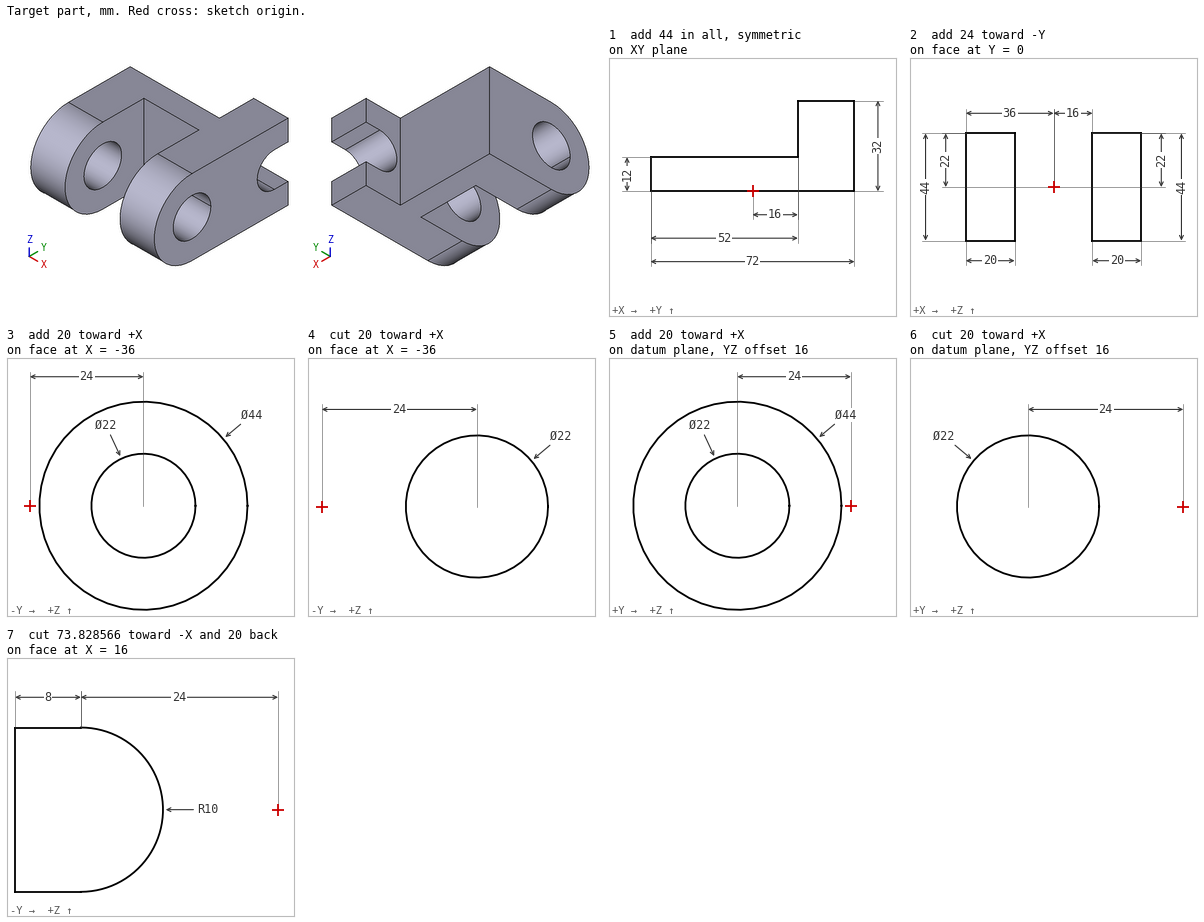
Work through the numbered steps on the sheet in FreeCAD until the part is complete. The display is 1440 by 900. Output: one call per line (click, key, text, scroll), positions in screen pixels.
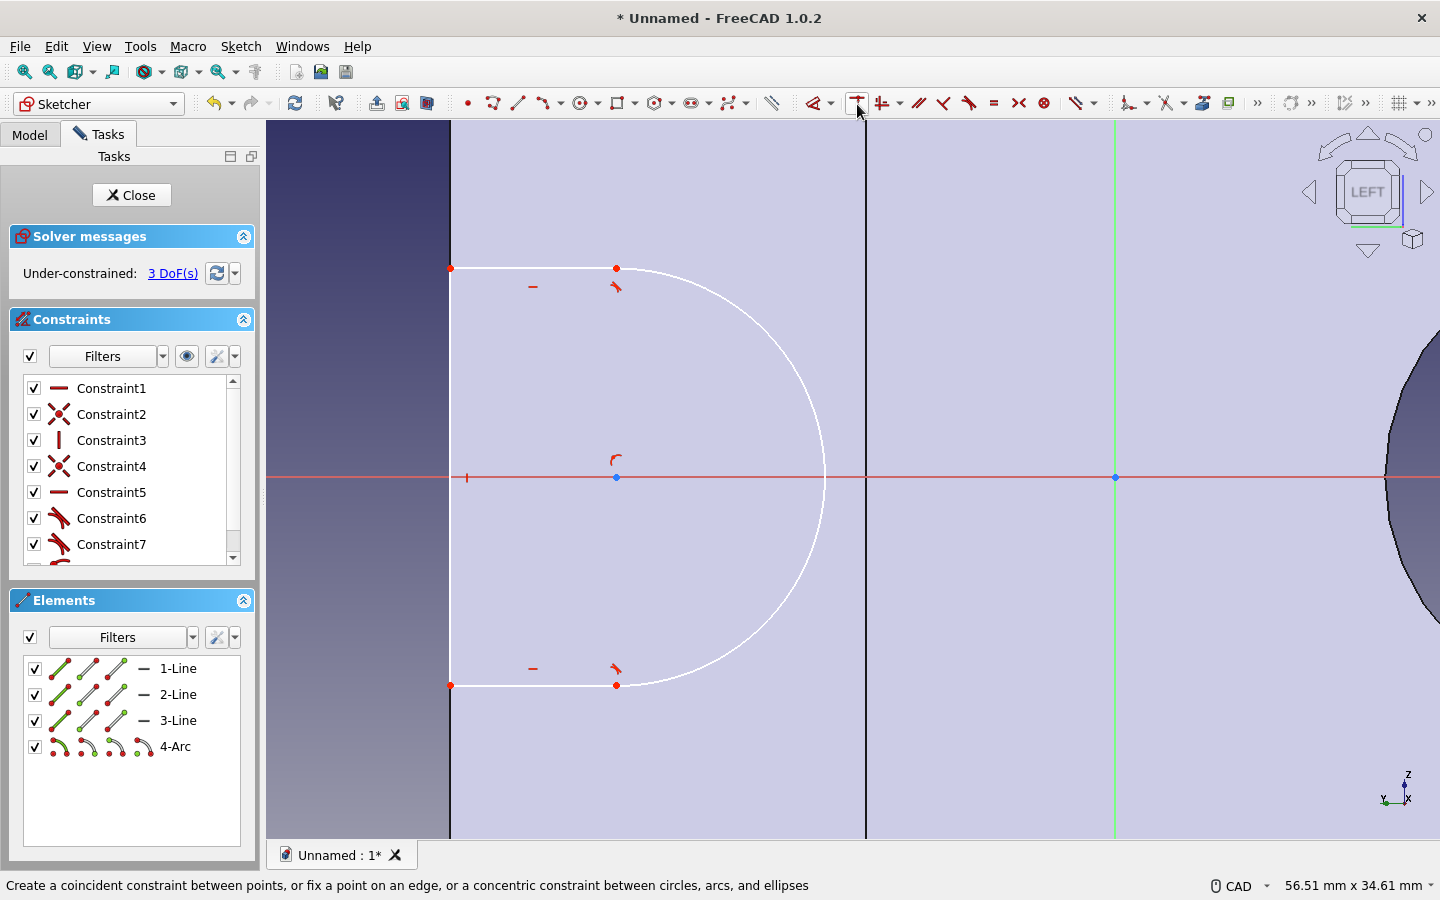
click(812, 104)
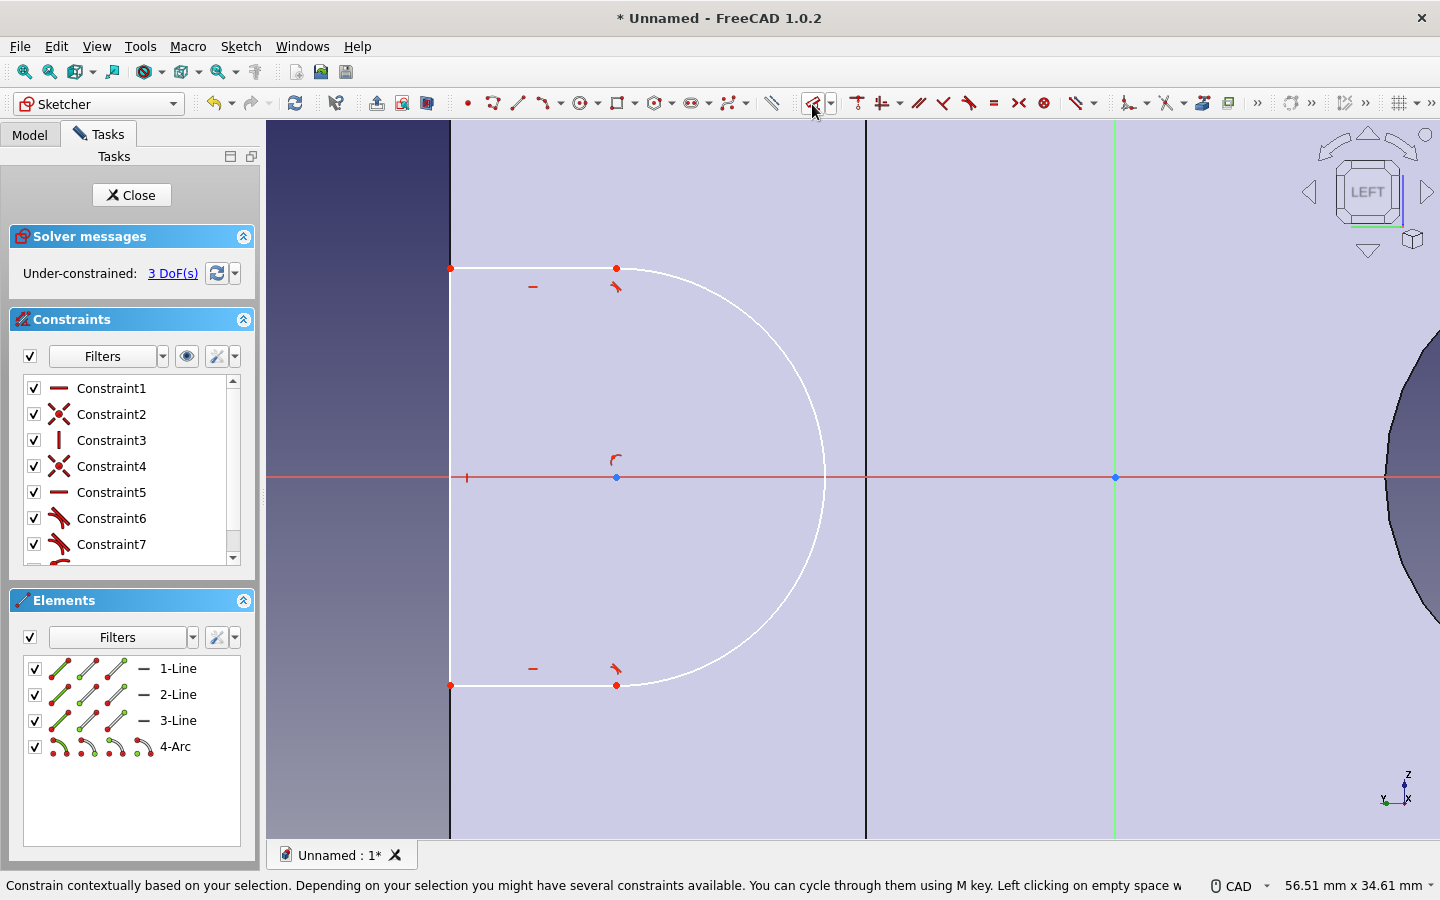
click(785, 600)
click(811, 619)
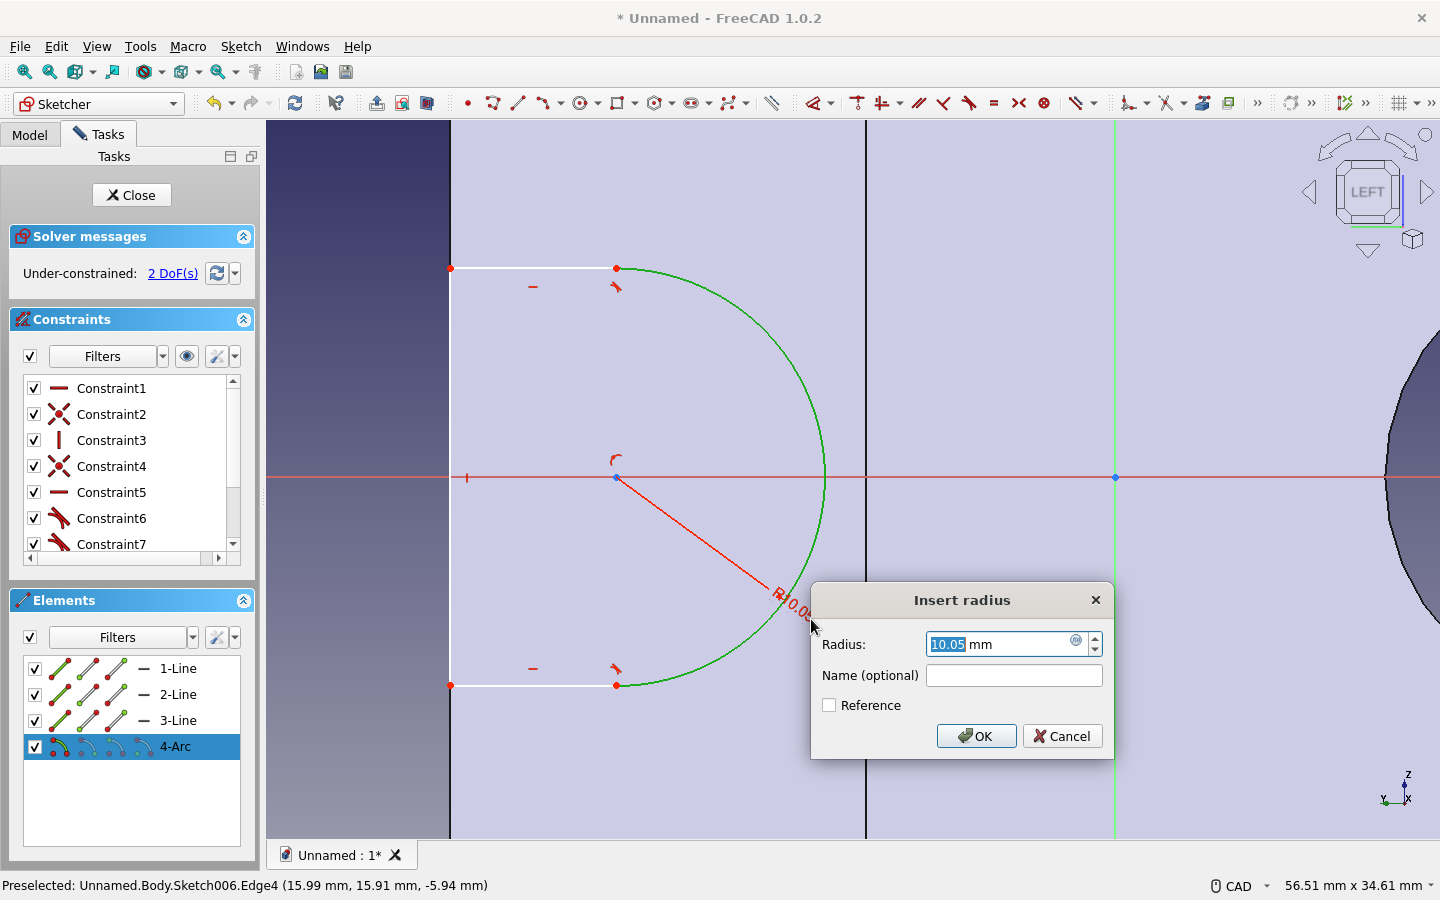
text(10)
key(Return)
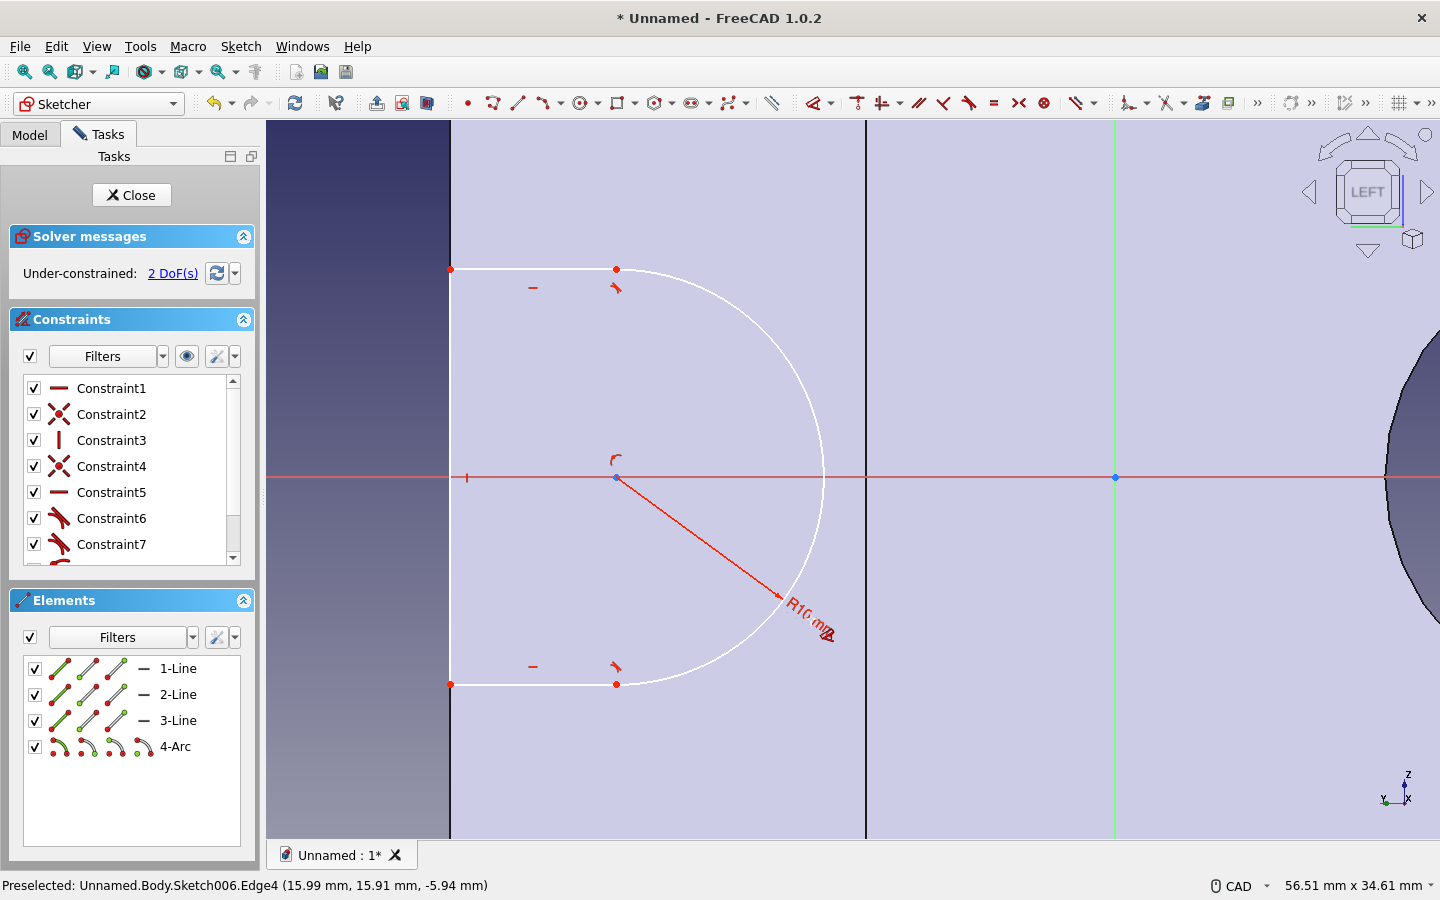
click(566, 269)
click(533, 235)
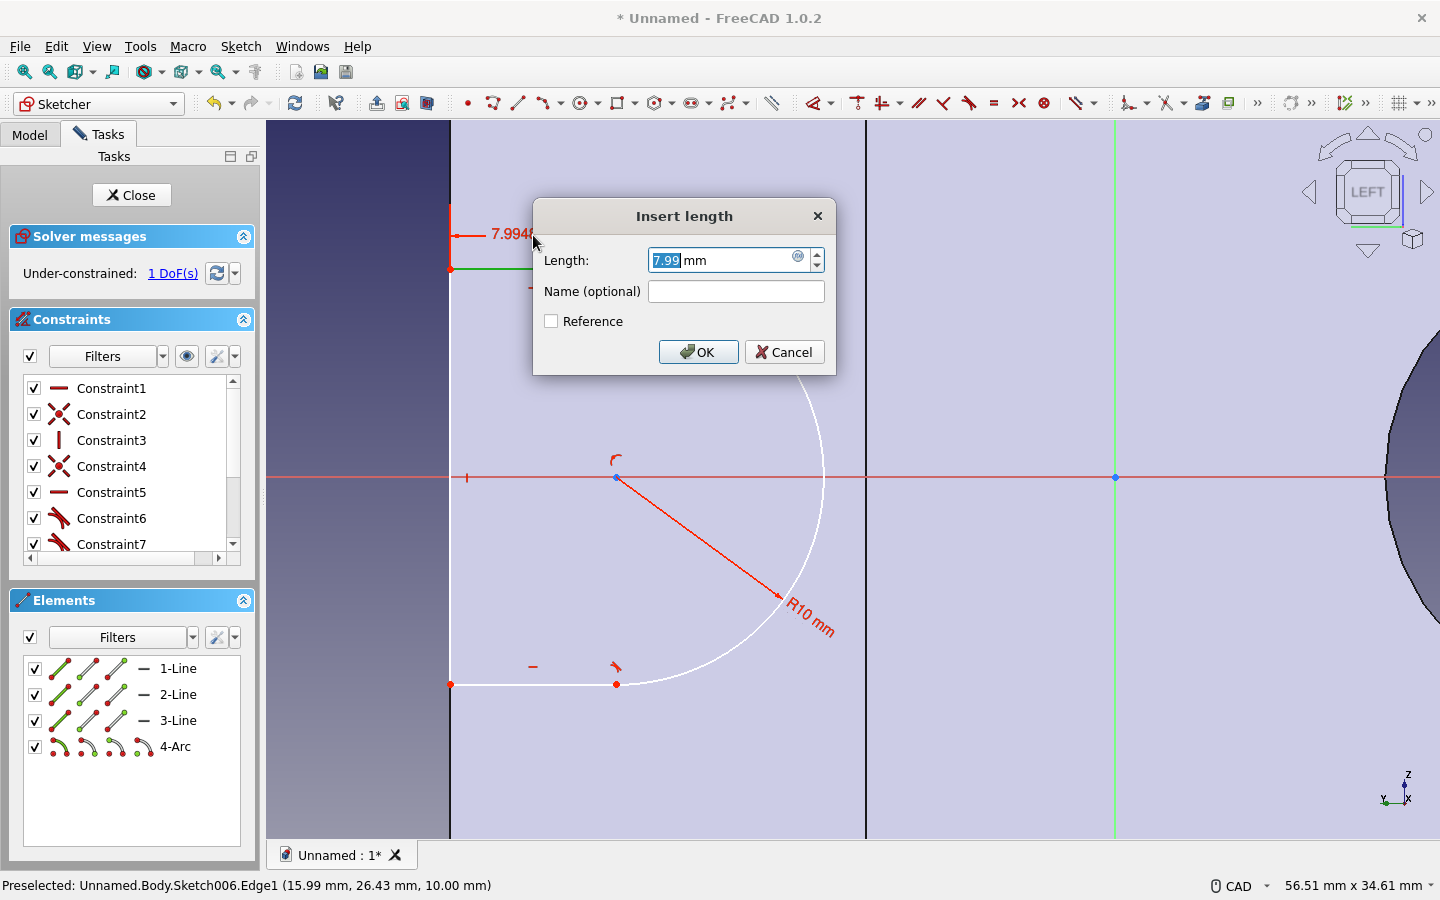
text(8)
key(Return)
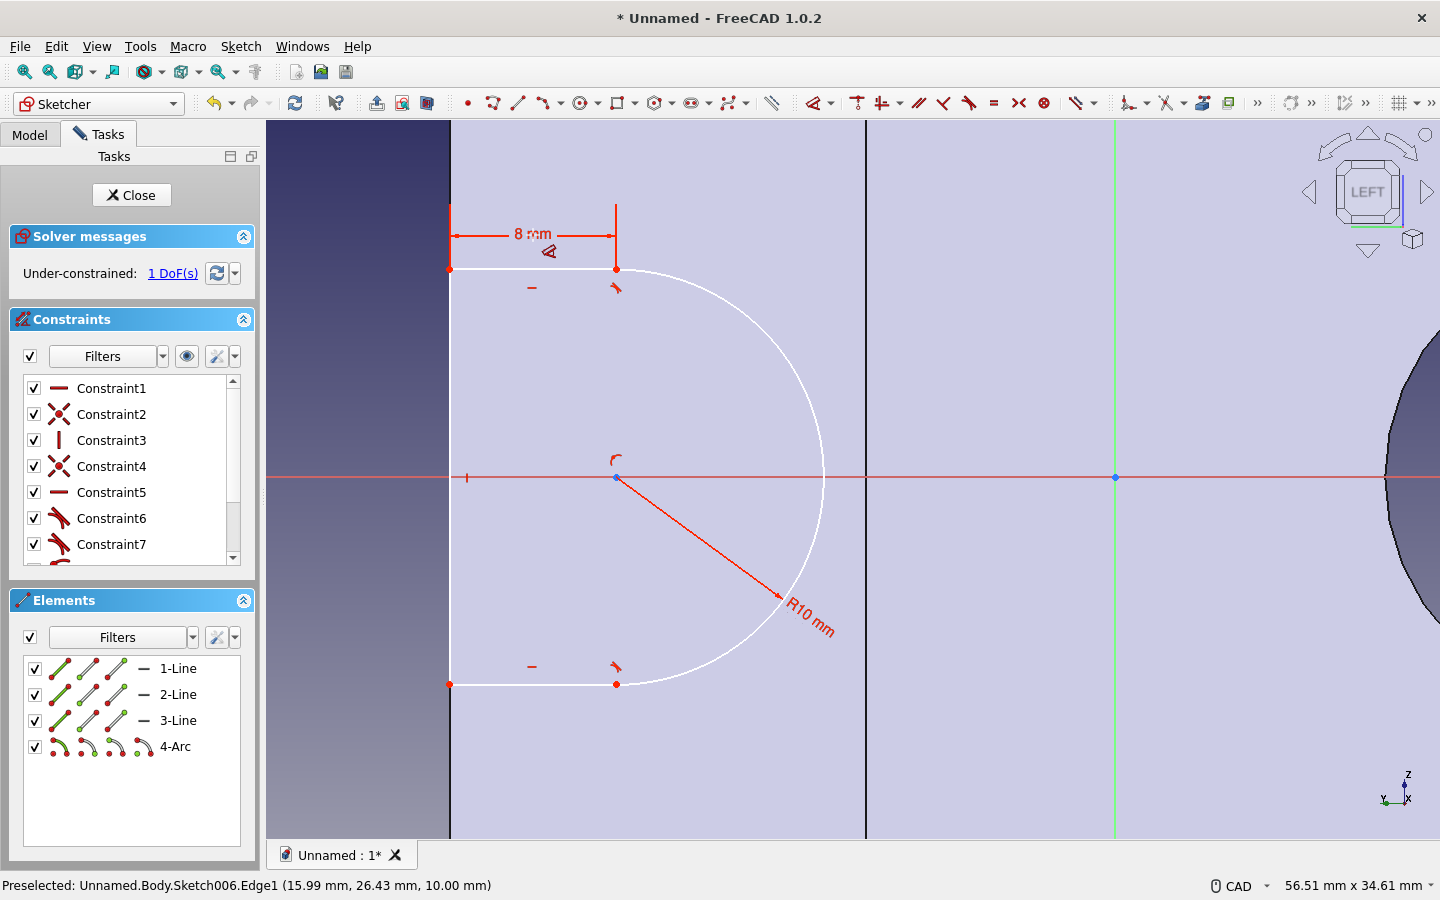
click(616, 269)
click(866, 235)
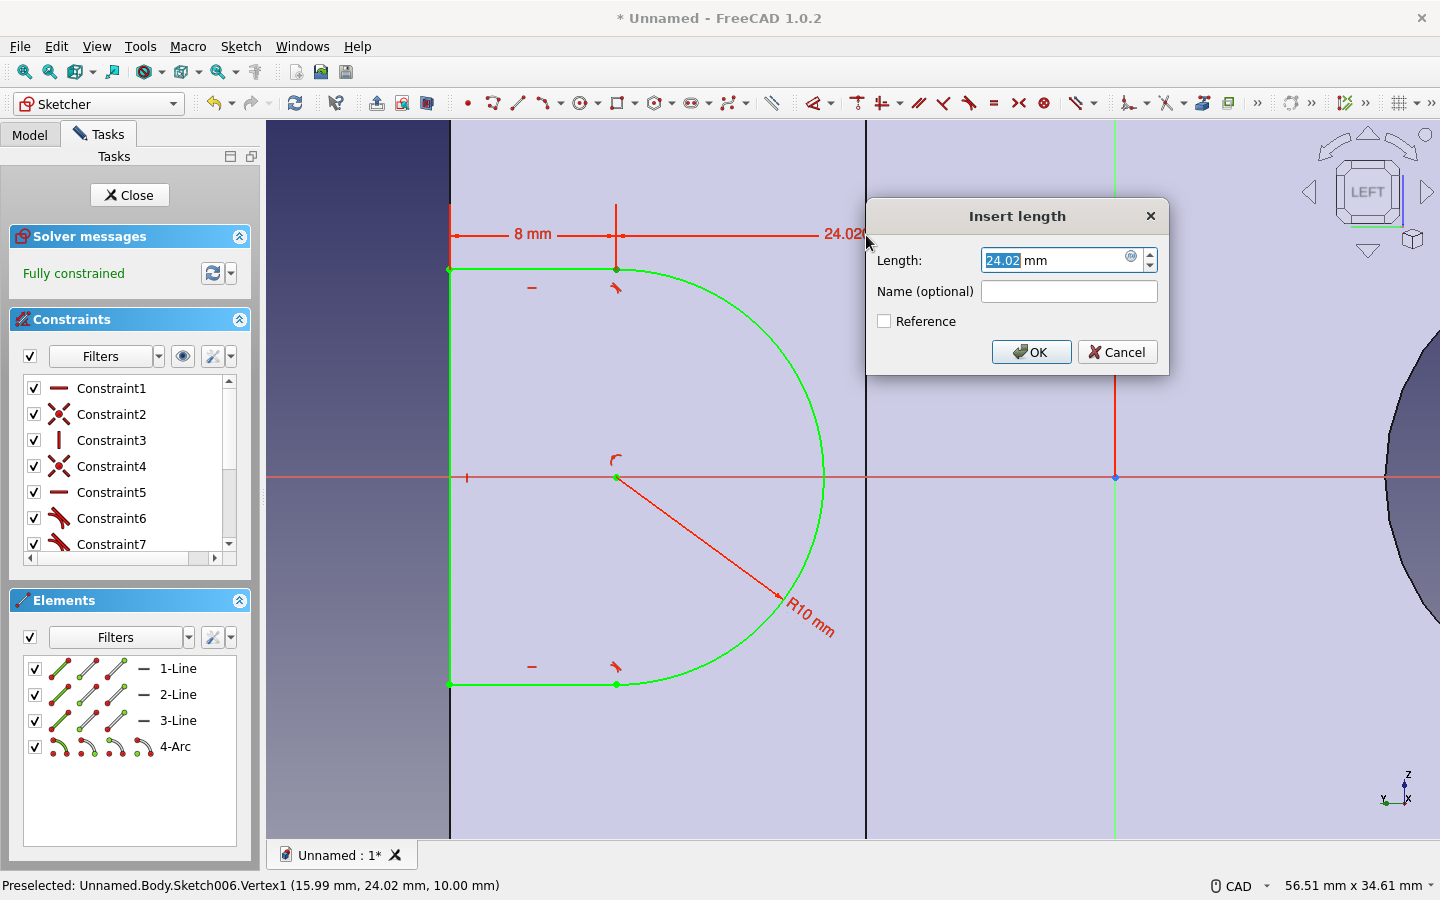
text(24)
key(Return)
key(Escape)